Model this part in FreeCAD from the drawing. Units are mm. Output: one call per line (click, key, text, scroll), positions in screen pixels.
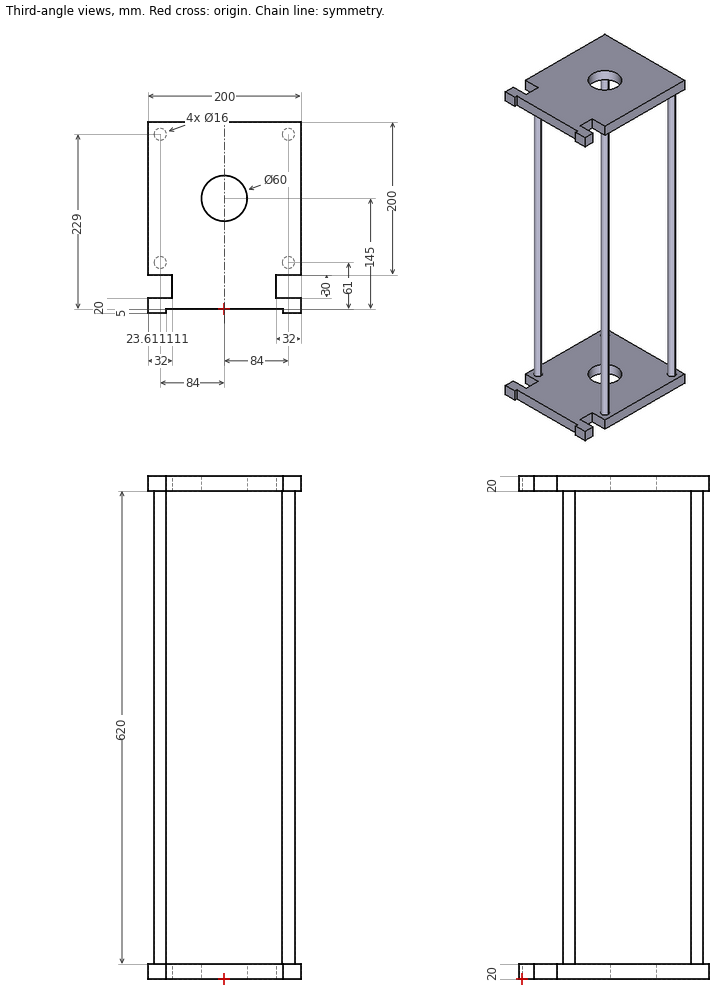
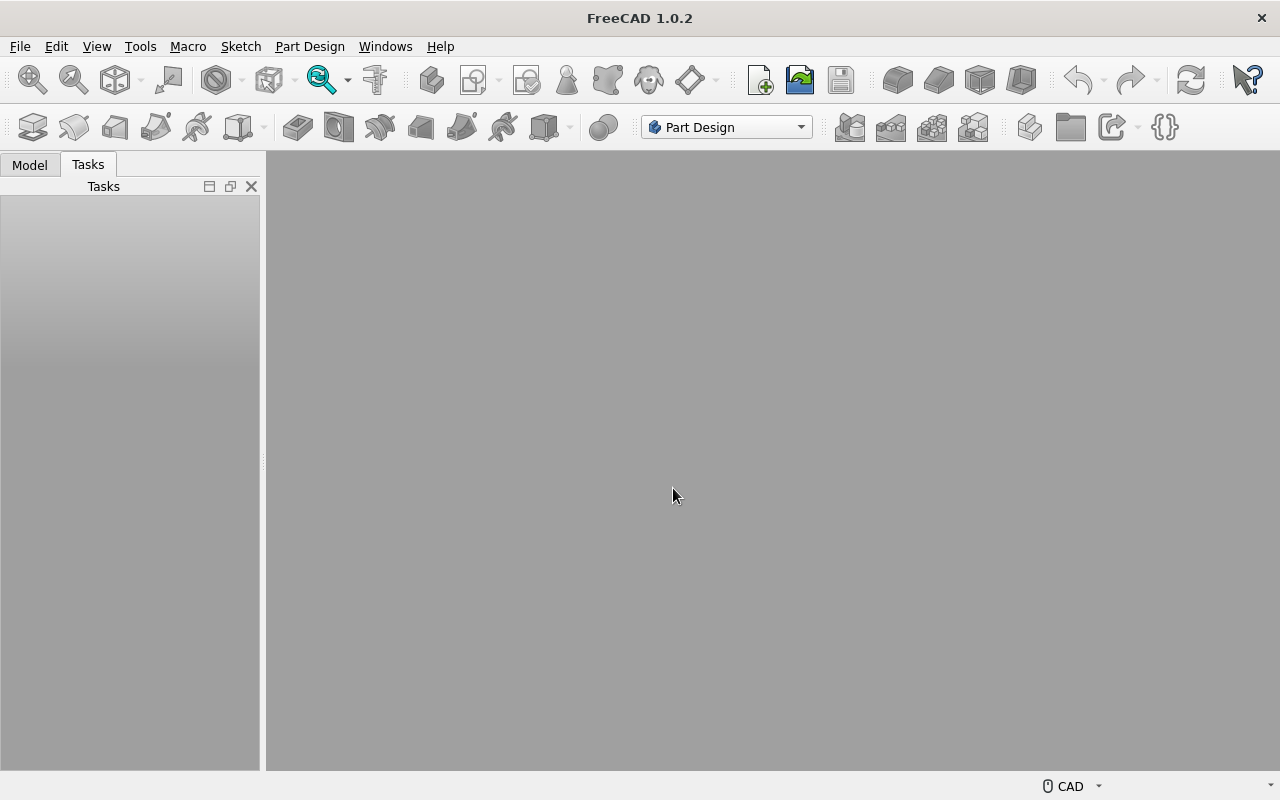
click(759, 80)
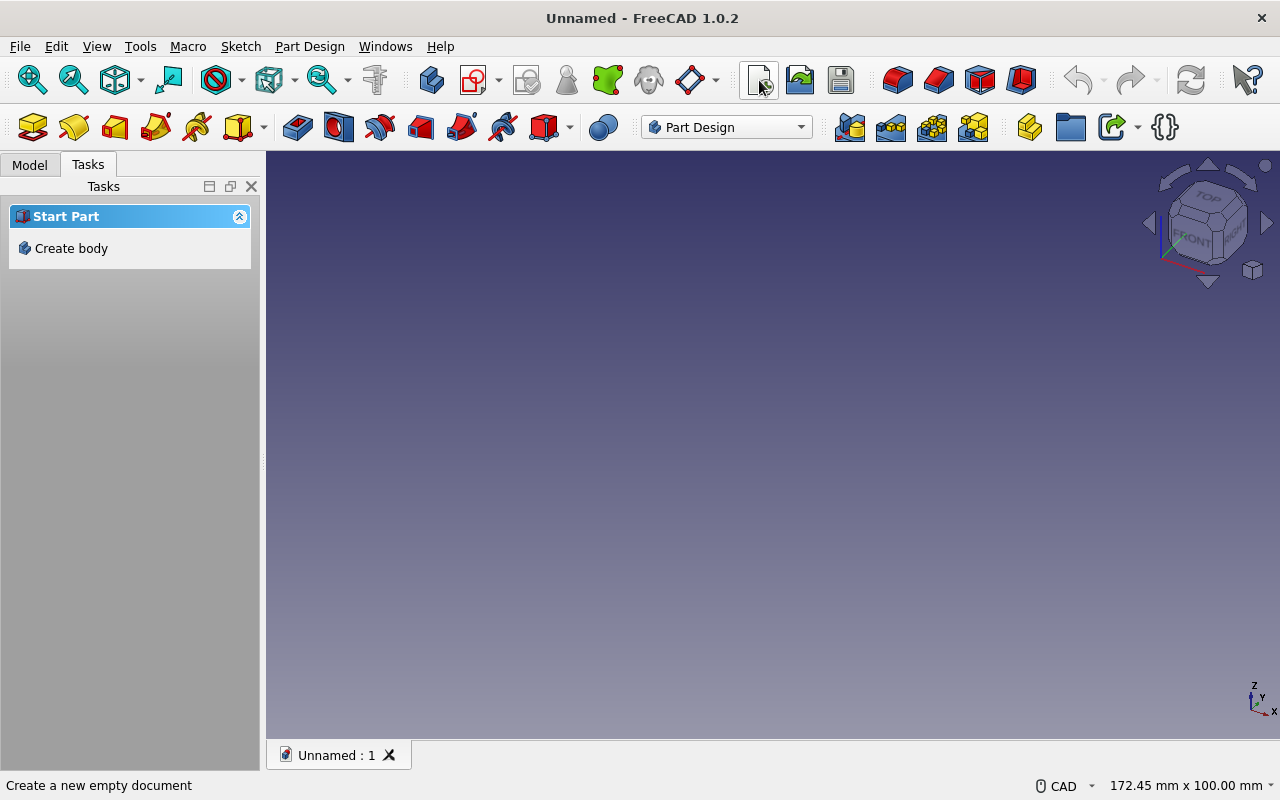
click(472, 80)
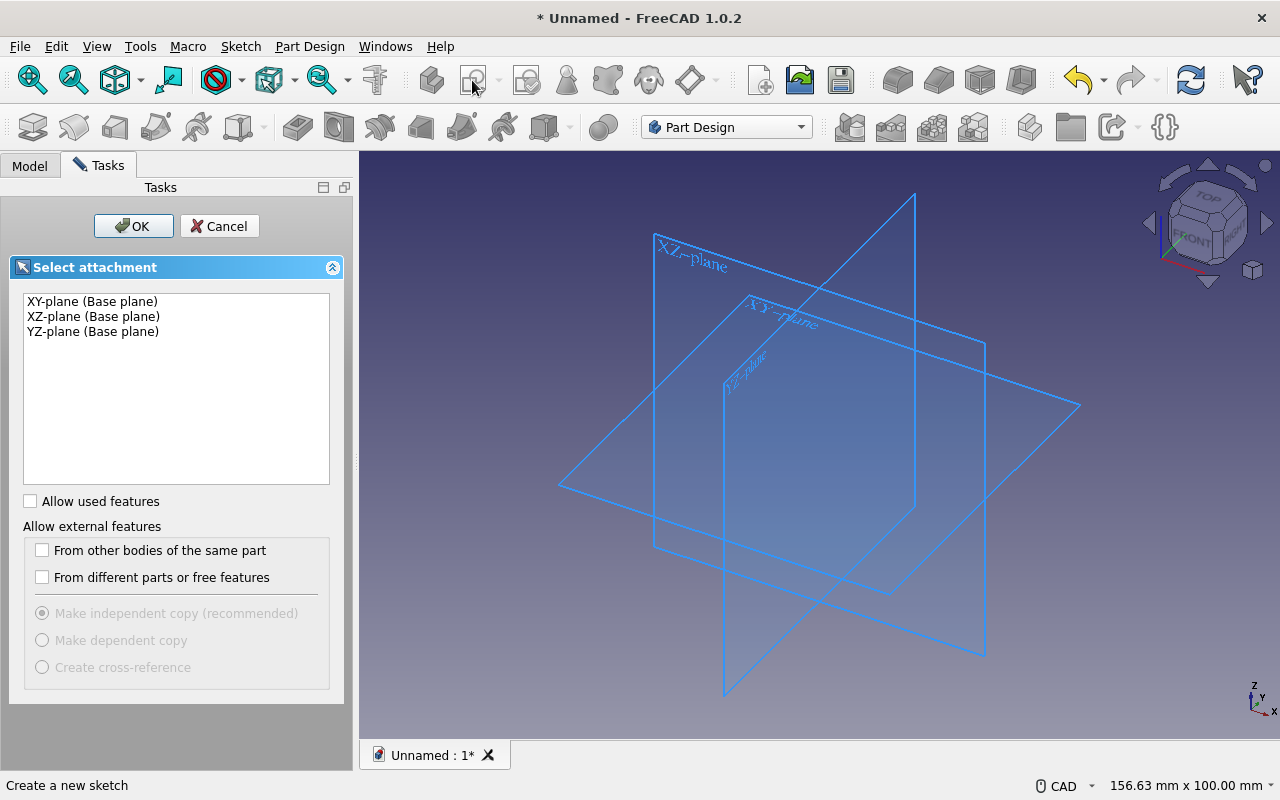
click(84, 302)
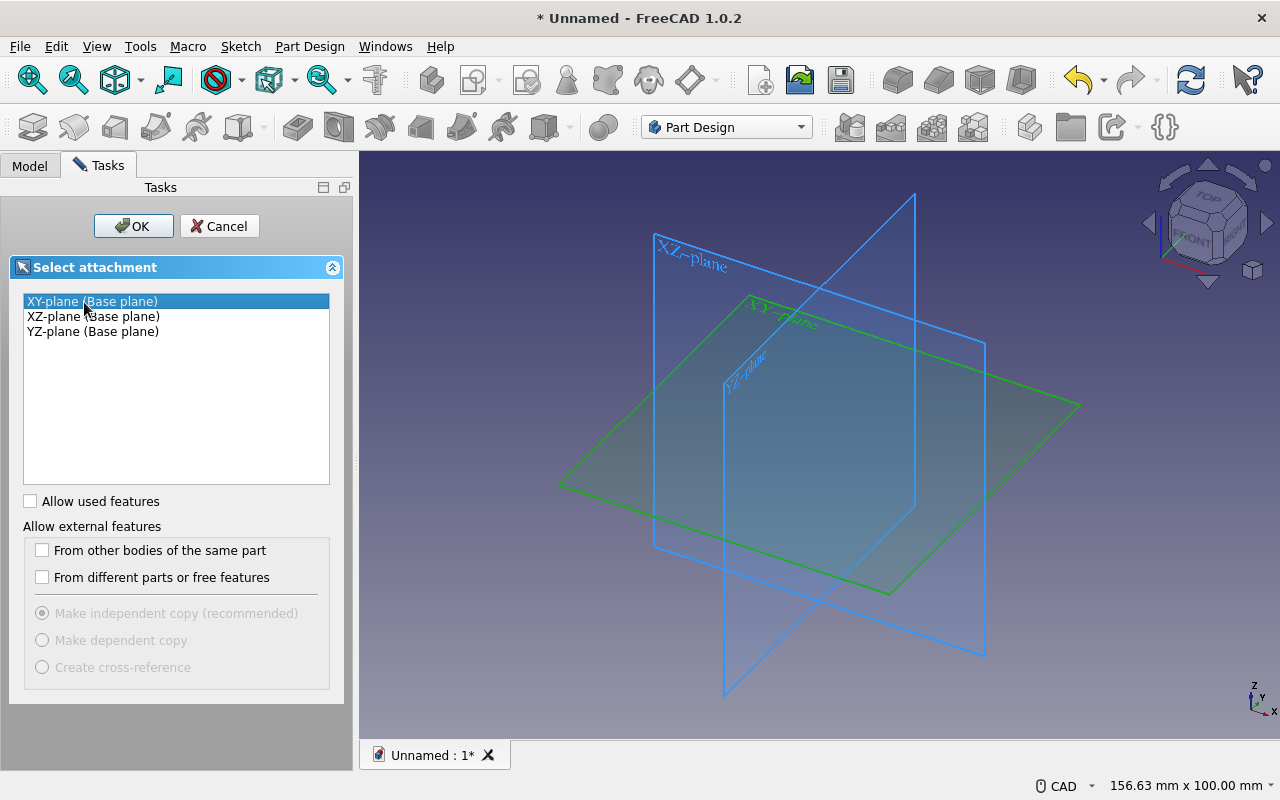
click(134, 226)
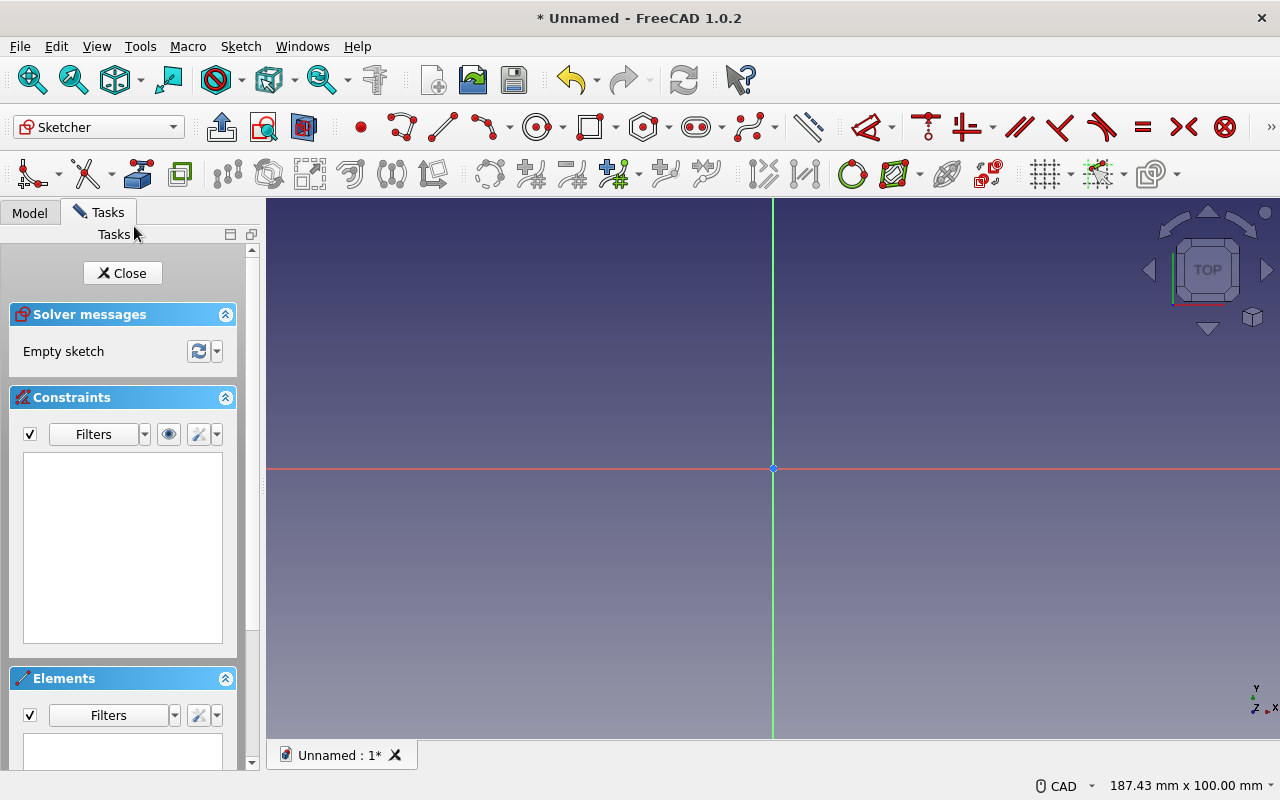
scroll(682, 681, down, 7)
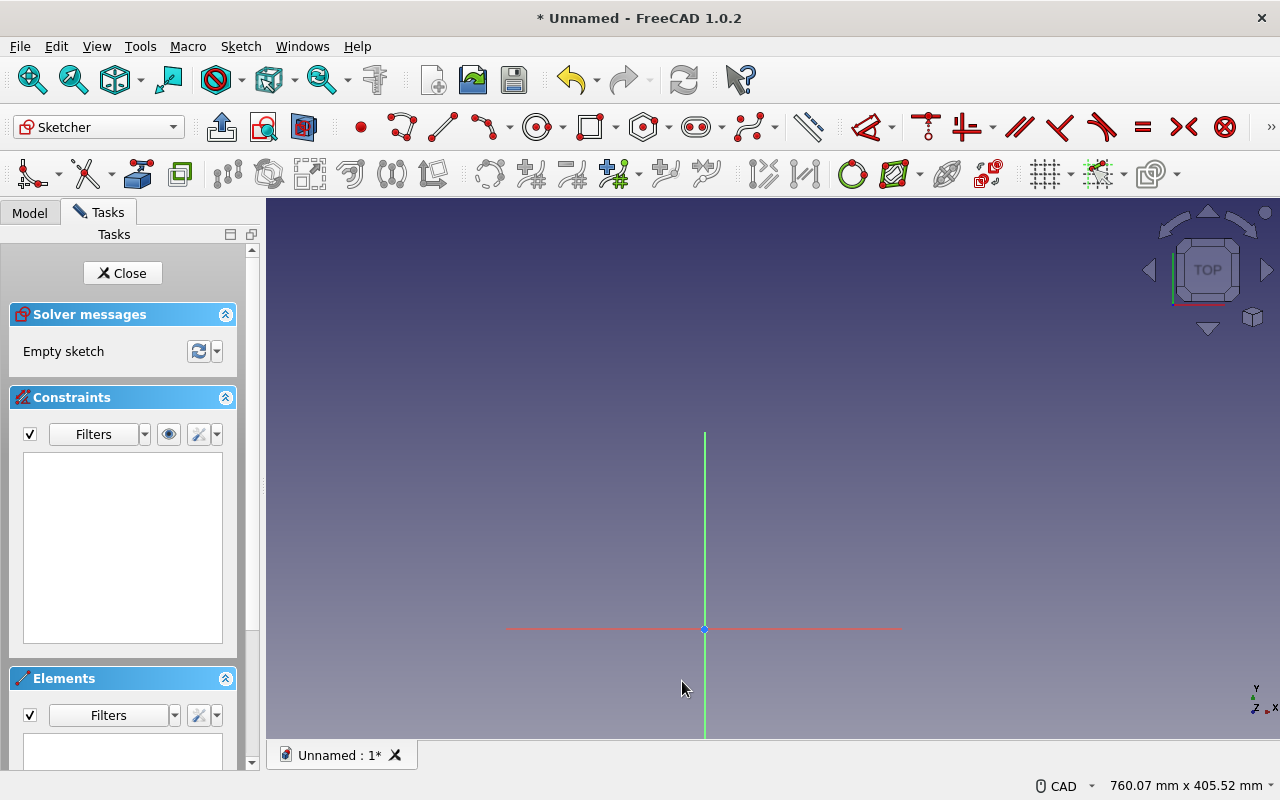
click(402, 128)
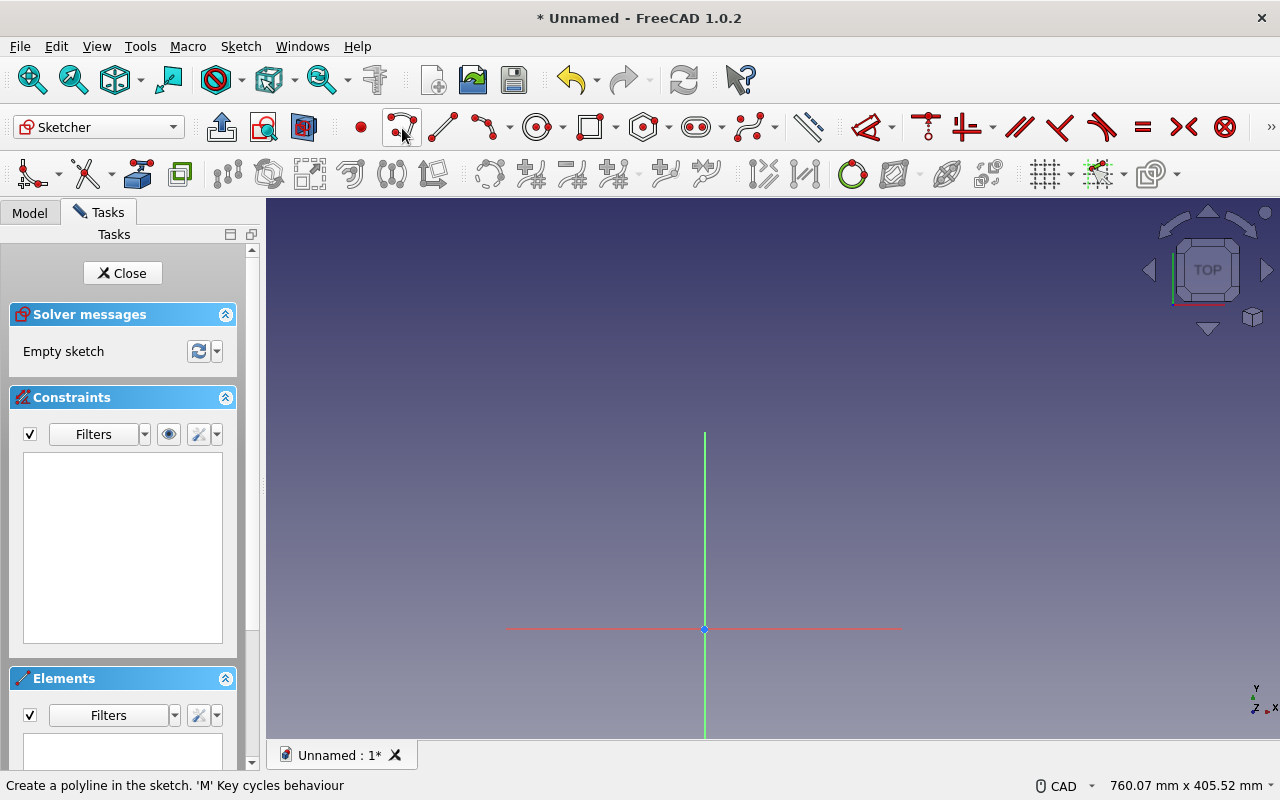
click(795, 609)
click(795, 569)
click(838, 569)
click(838, 302)
click(571, 302)
click(571, 569)
click(614, 569)
click(614, 609)
click(571, 609)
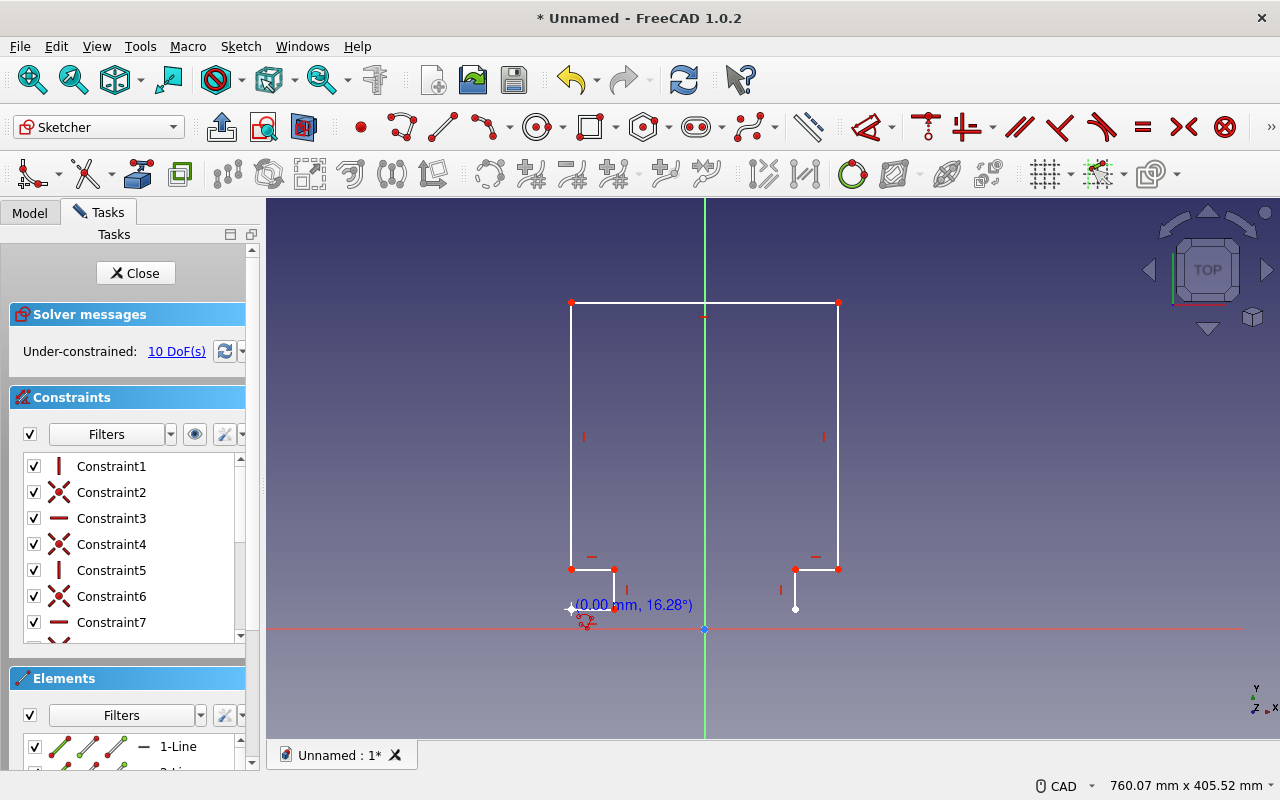
scroll(571, 636, up, 5)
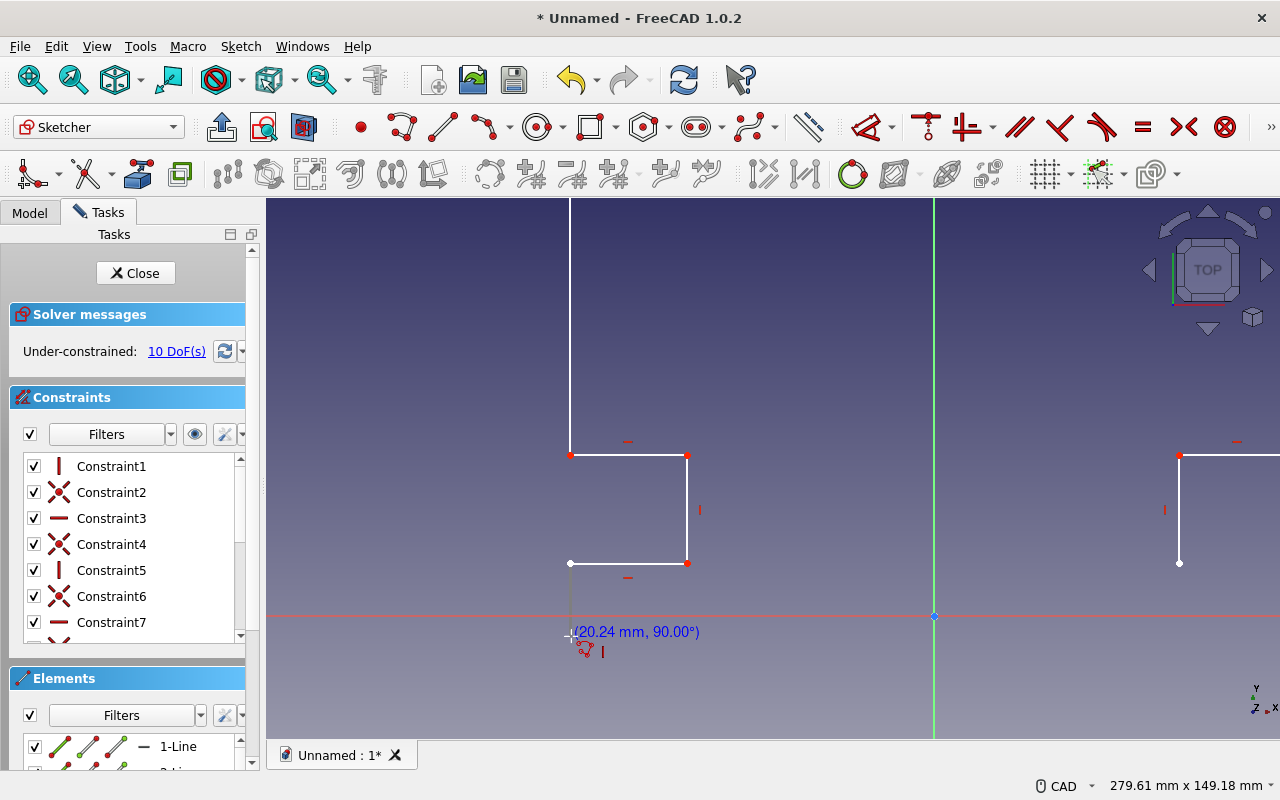
click(570, 634)
click(657, 634)
click(657, 616)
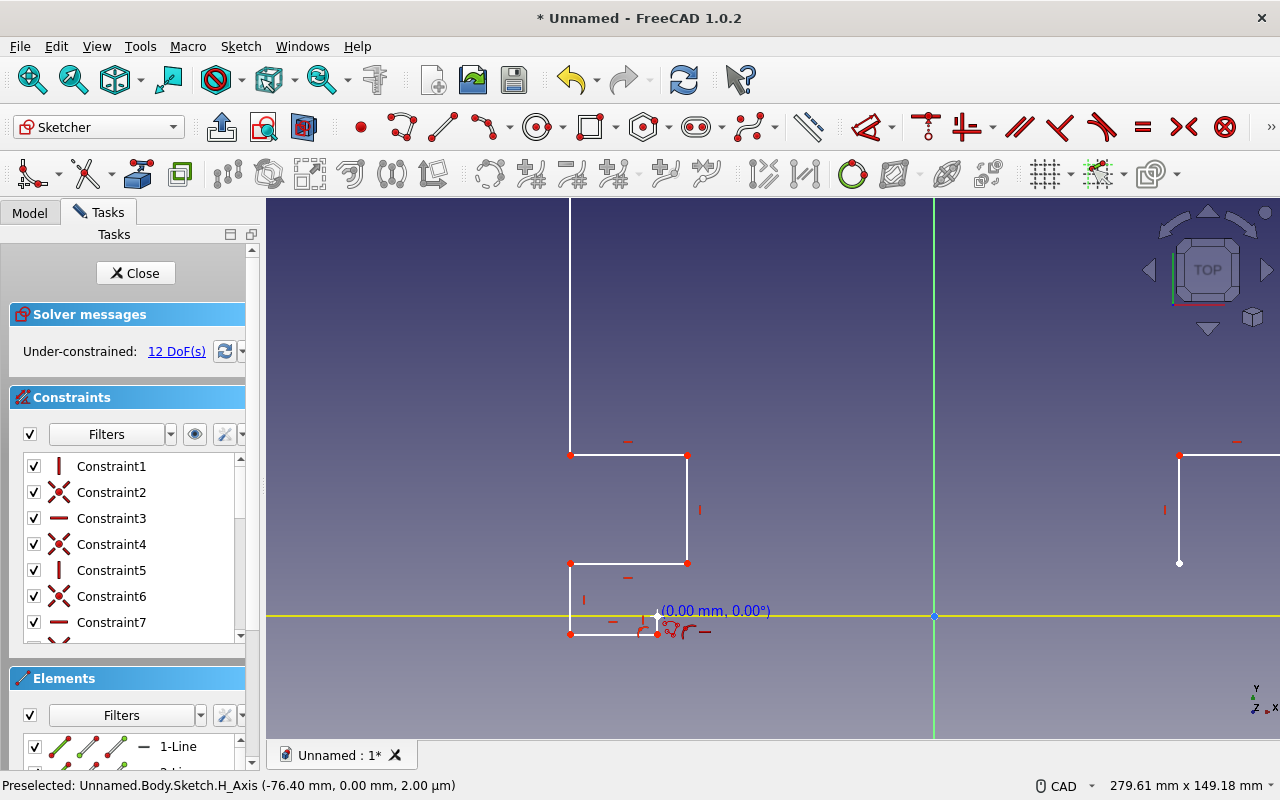
scroll(571, 636, down, 5)